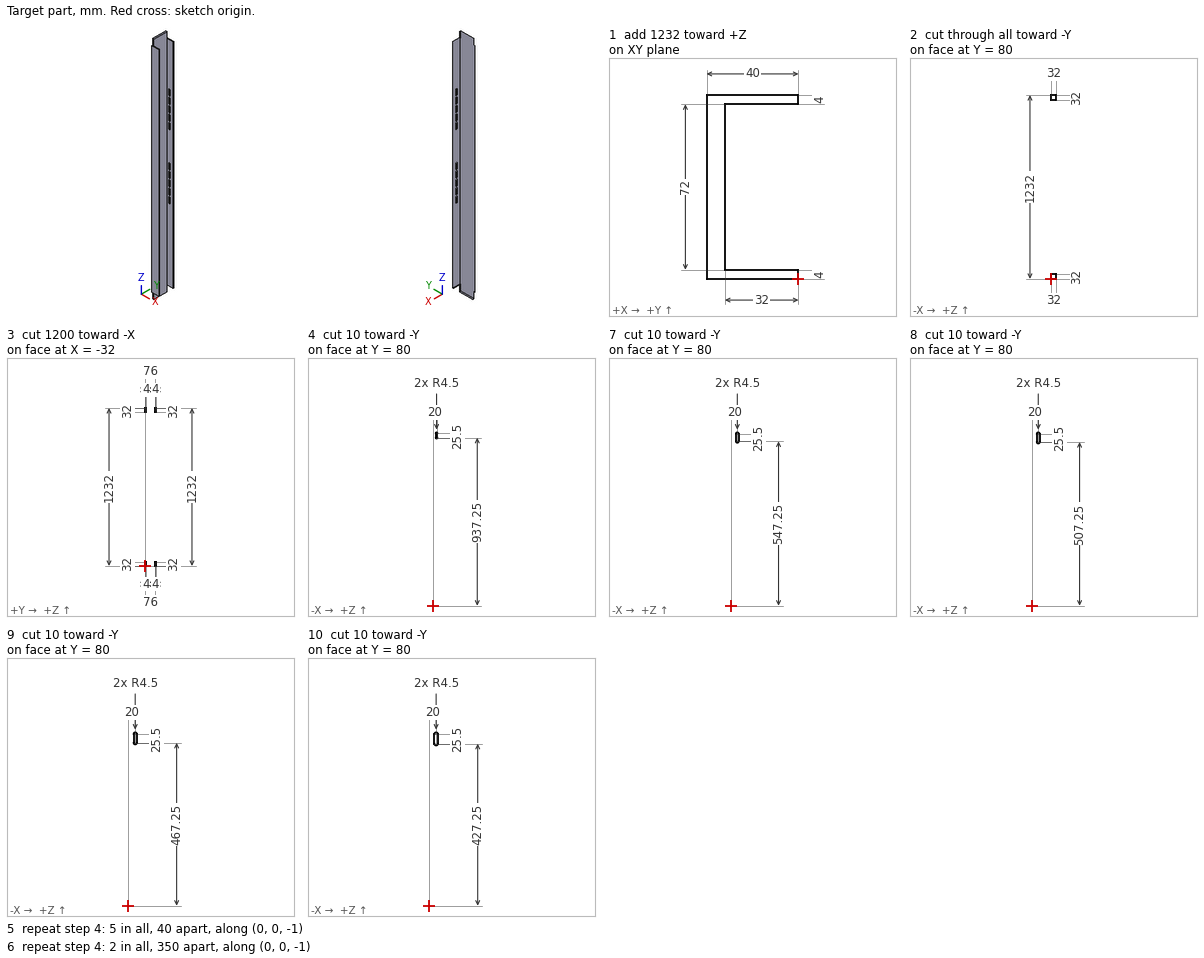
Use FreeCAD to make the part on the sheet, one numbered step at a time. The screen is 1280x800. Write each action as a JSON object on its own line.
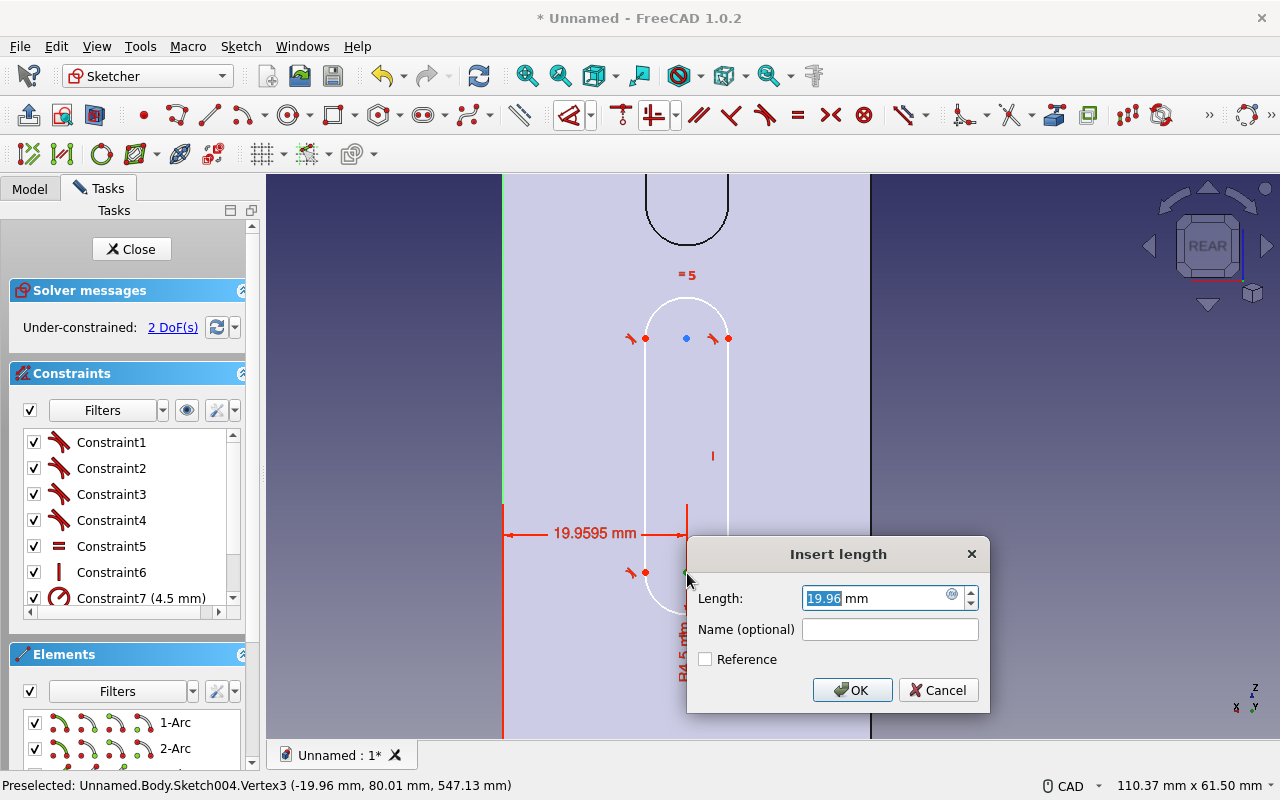
{"action": "type", "text": "20"}
{"action": "key", "text": "Return"}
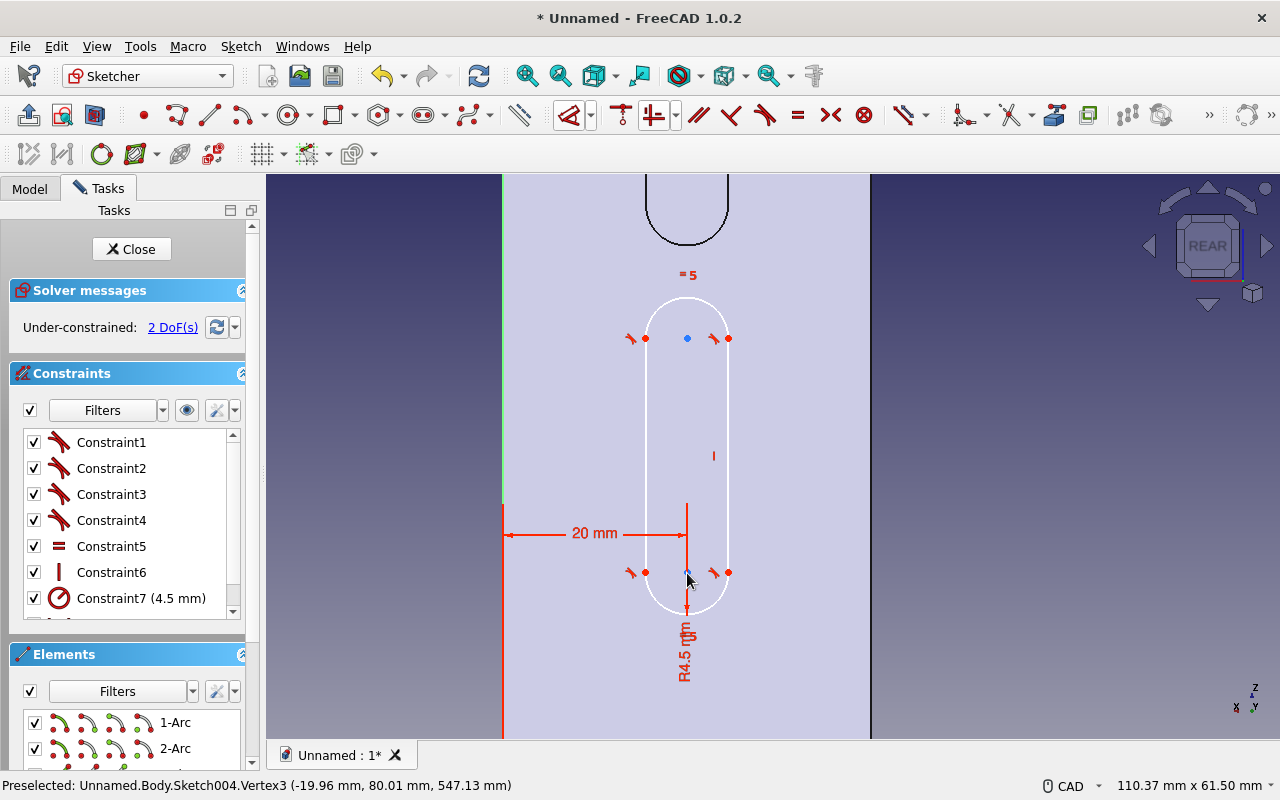
{"action": "left_click", "coordinate": [646, 503]}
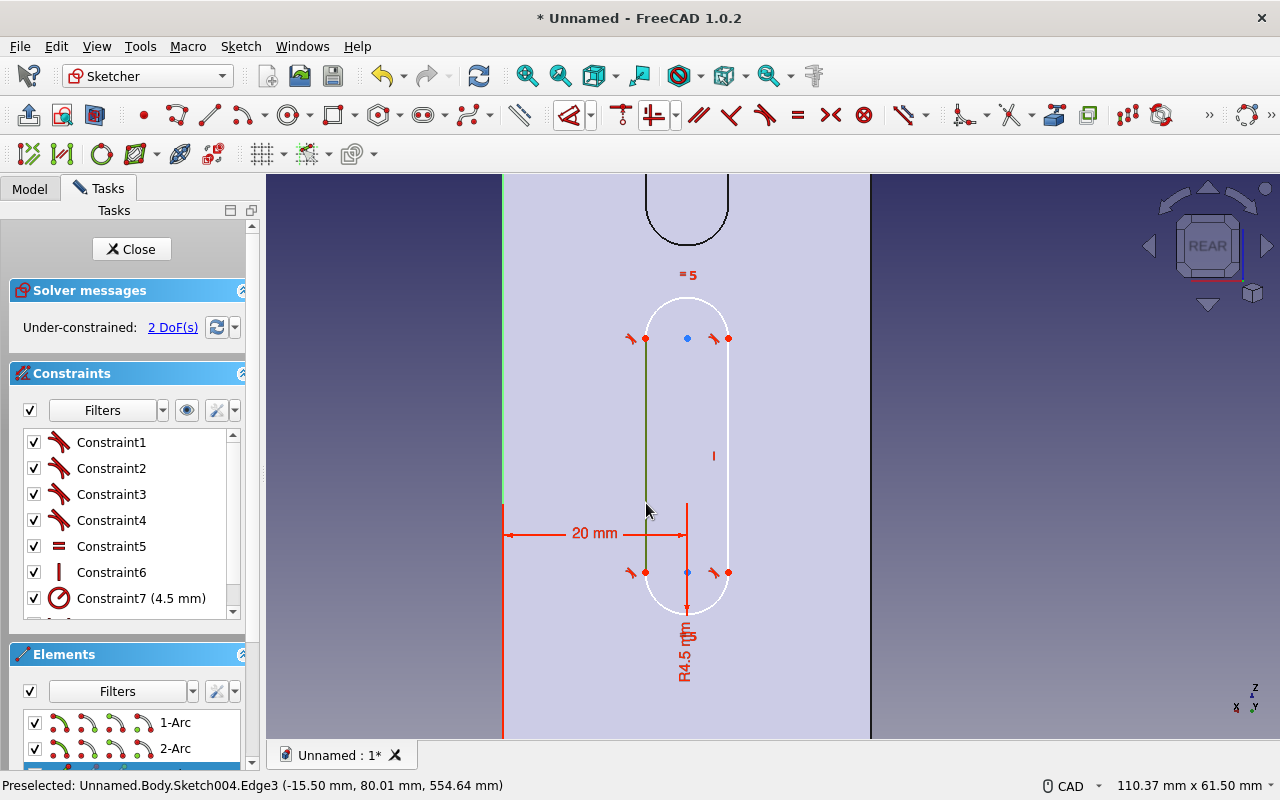
{"action": "left_click", "coordinate": [590, 116]}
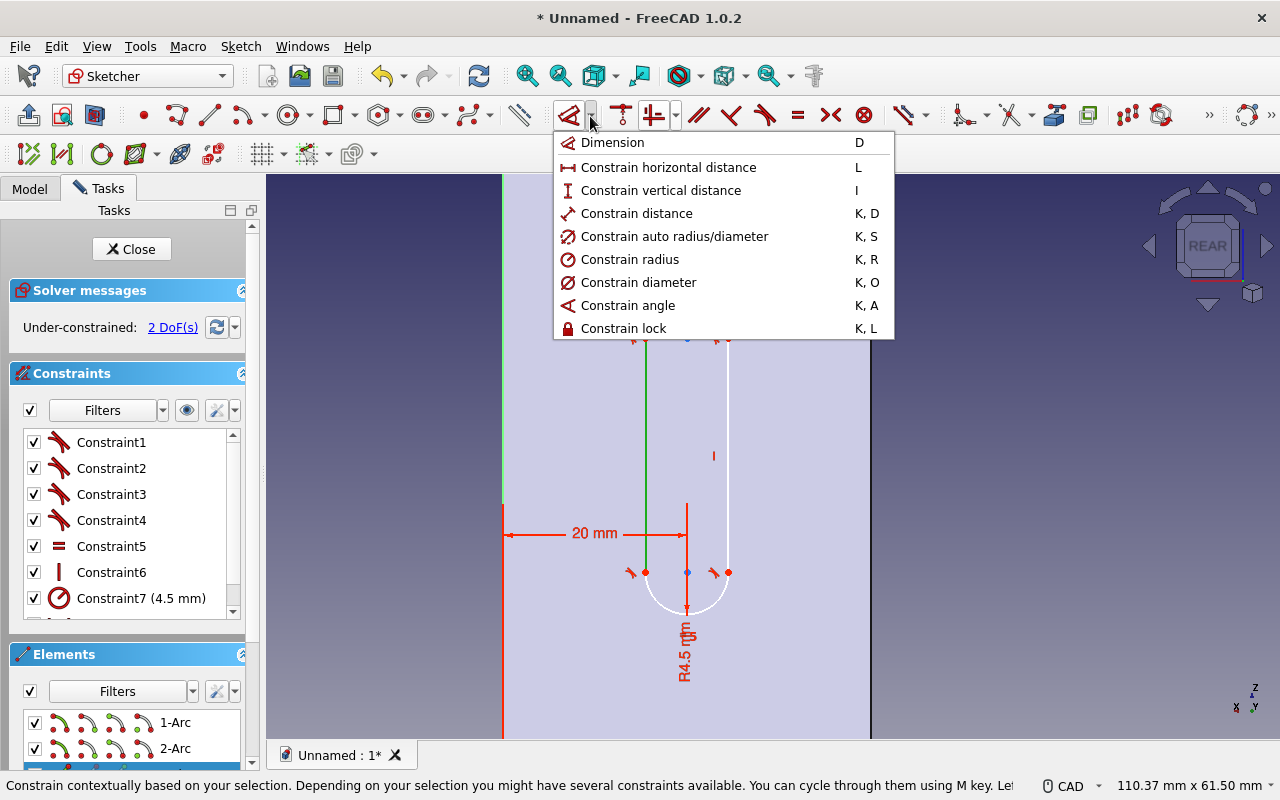
{"action": "left_click", "coordinate": [724, 190]}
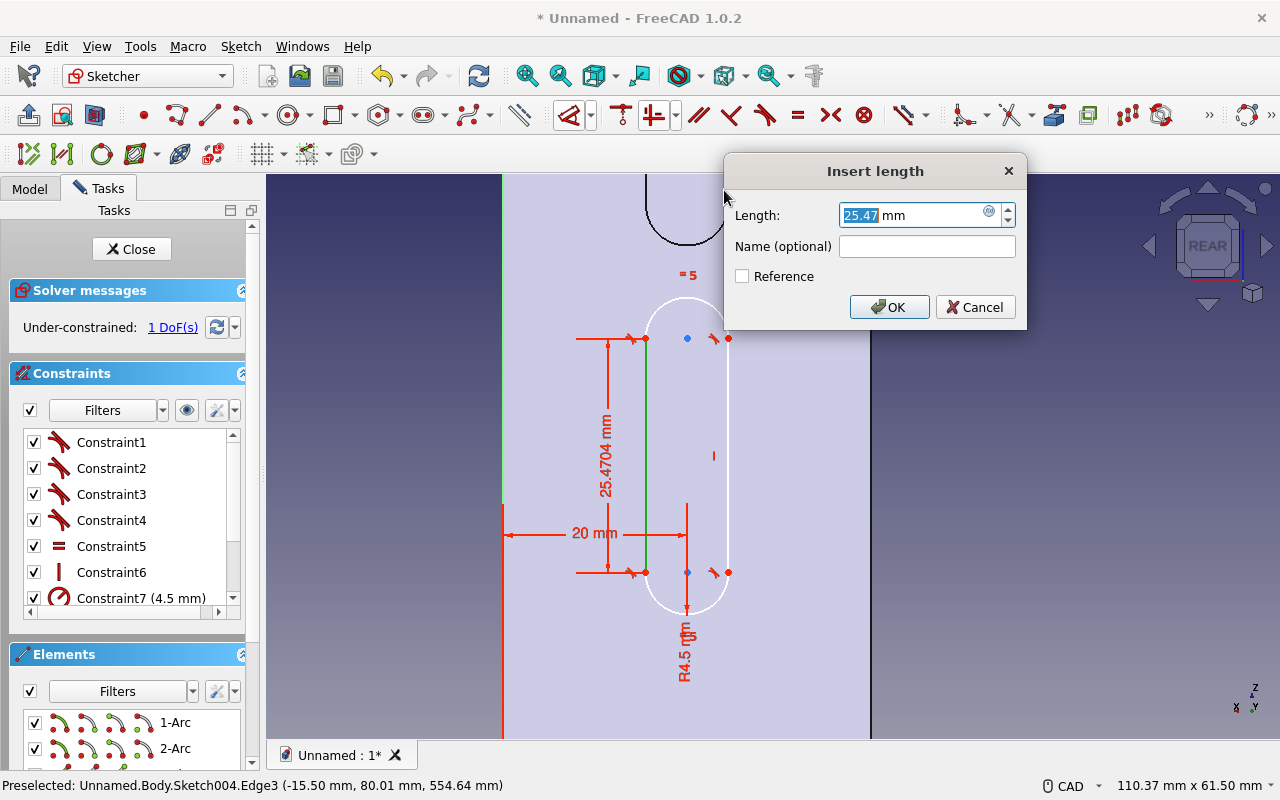
{"action": "type", "text": "25.5"}
{"action": "key", "text": "Return"}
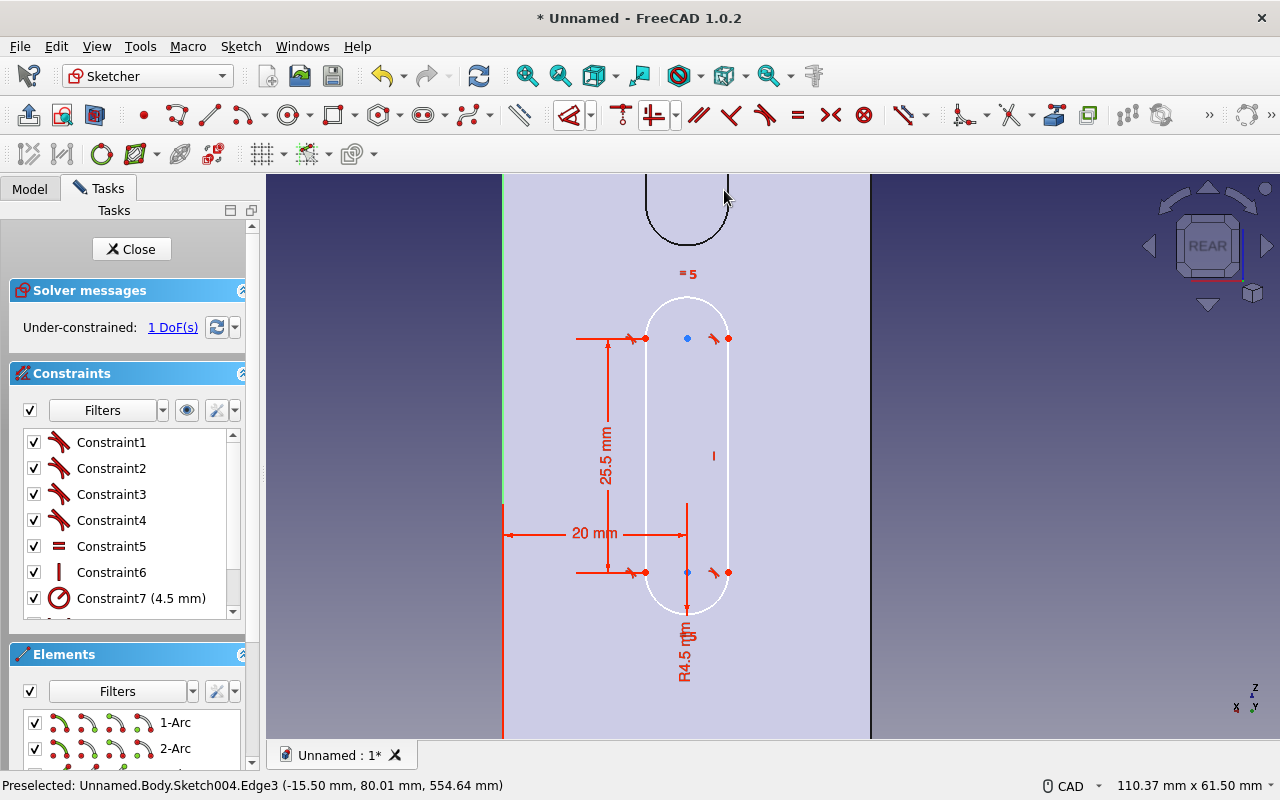
{"action": "left_click", "coordinate": [646, 573]}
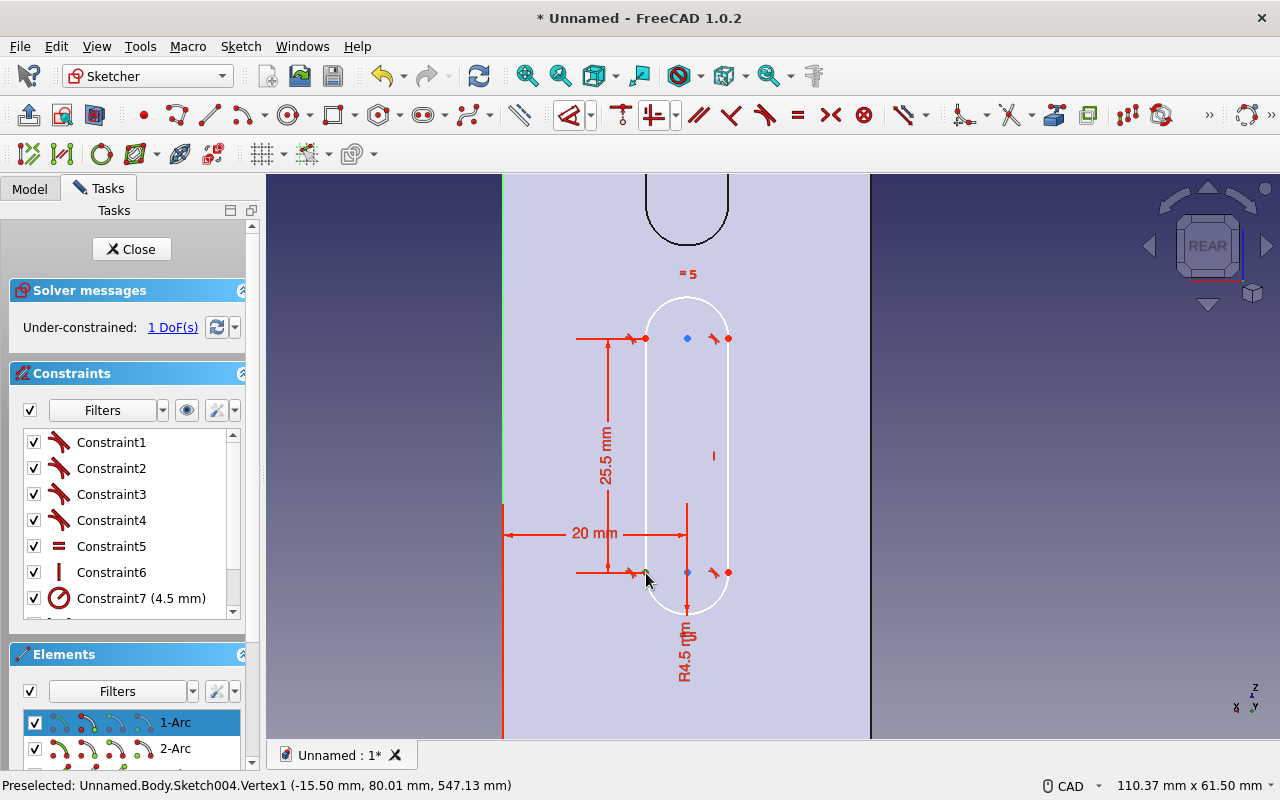
{"action": "key", "text": "i"}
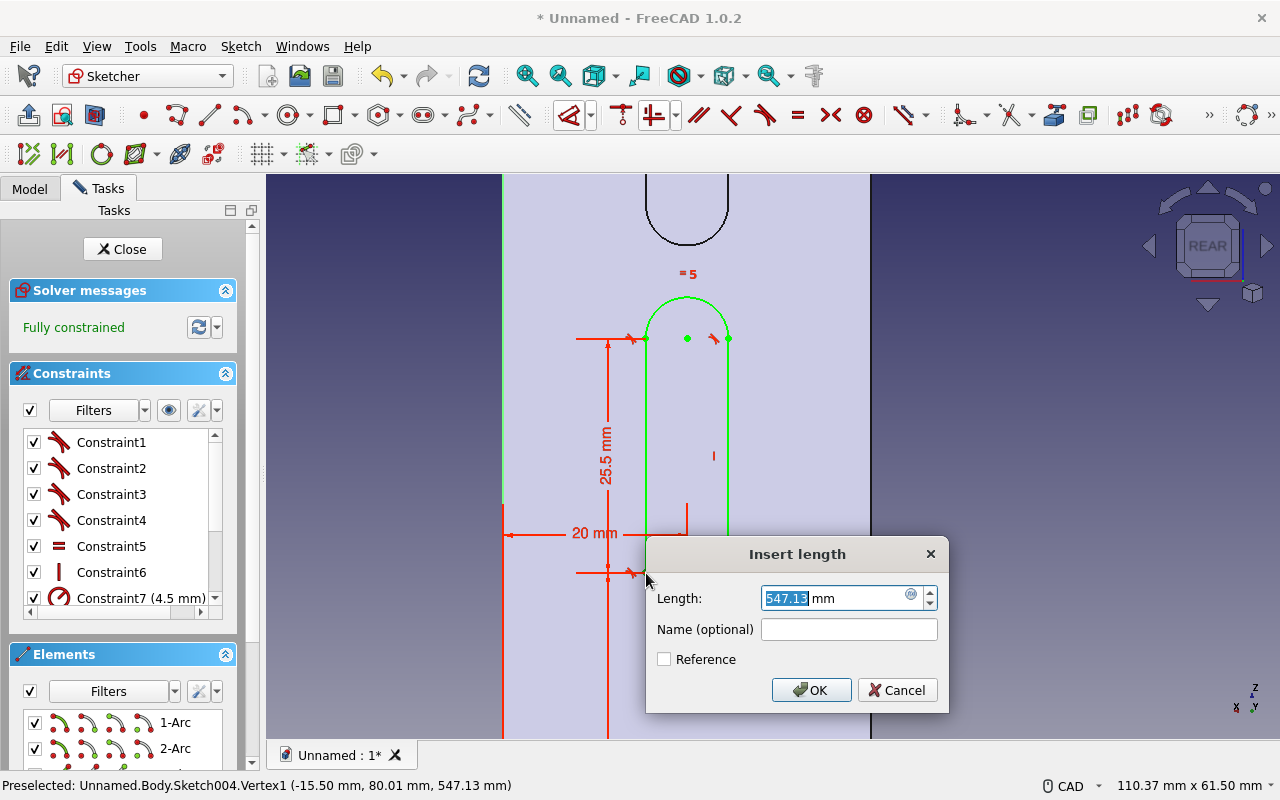
{"action": "type", "text": "547.25"}
{"action": "key", "text": "Return"}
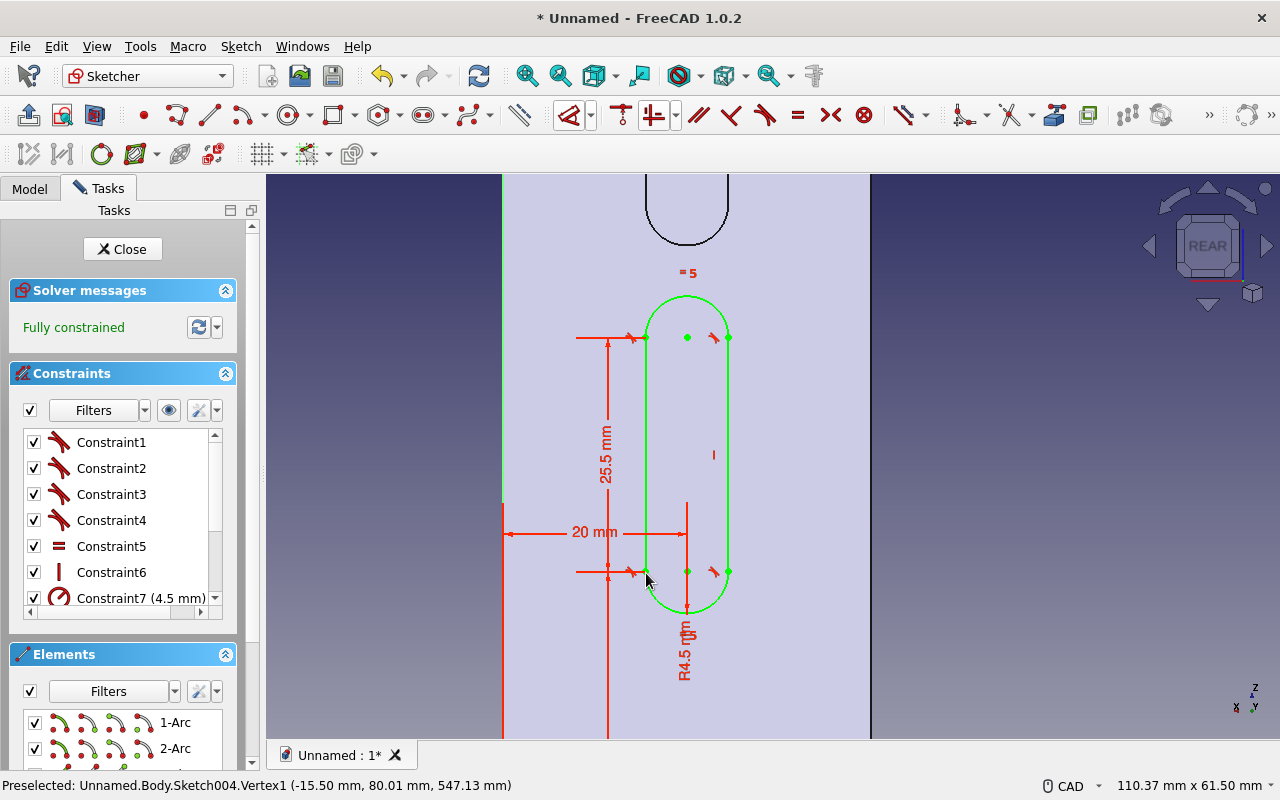
{"action": "left_click", "coordinate": [123, 249]}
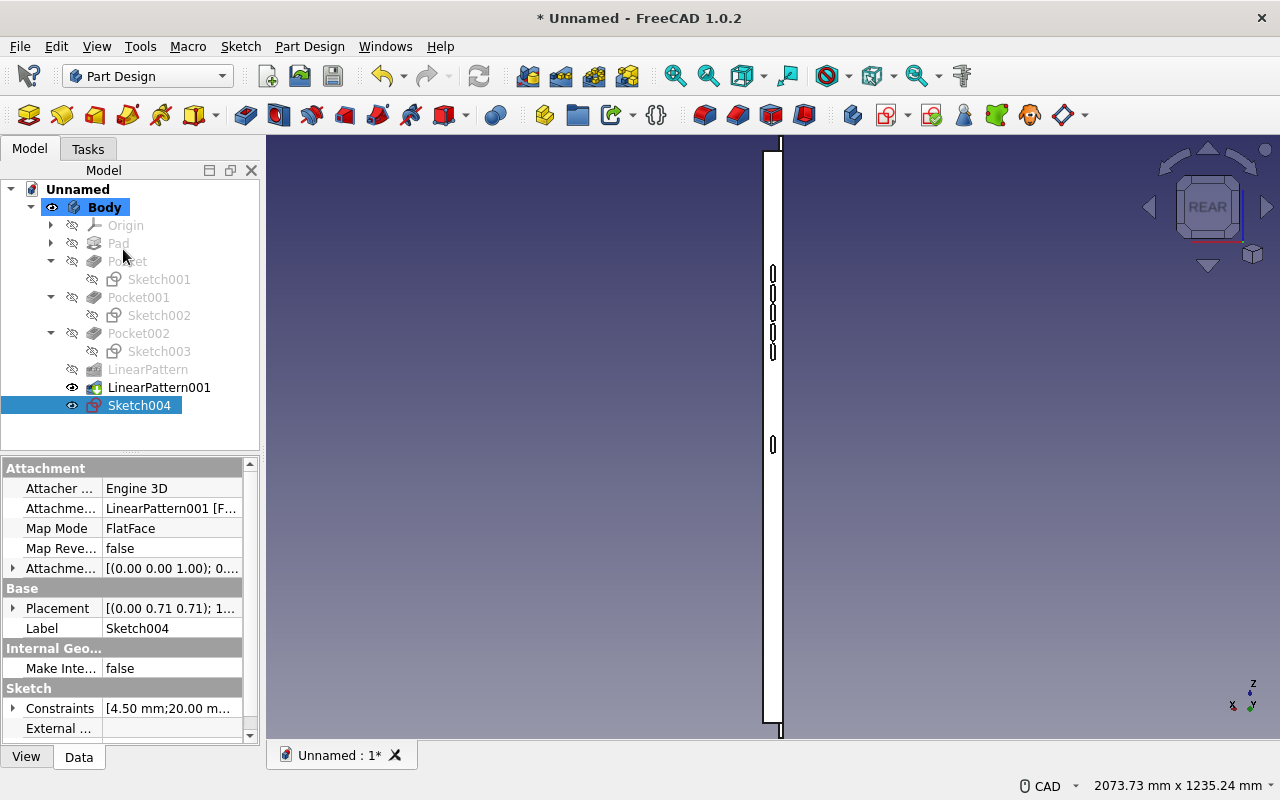
{"action": "left_click", "coordinate": [246, 116]}